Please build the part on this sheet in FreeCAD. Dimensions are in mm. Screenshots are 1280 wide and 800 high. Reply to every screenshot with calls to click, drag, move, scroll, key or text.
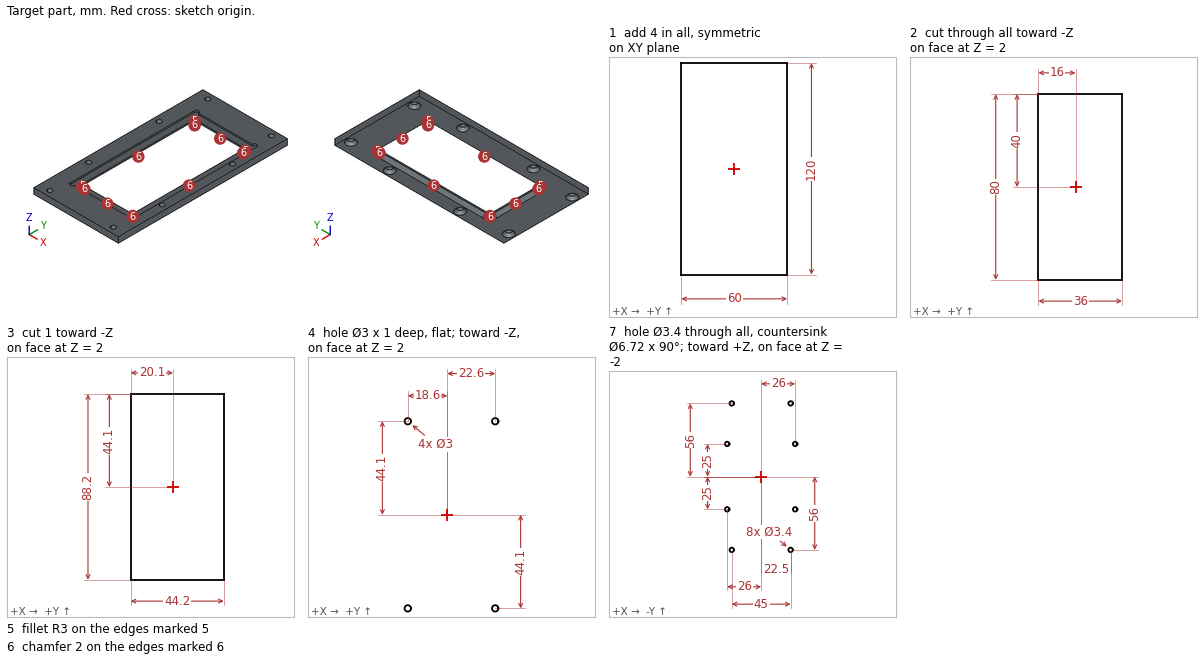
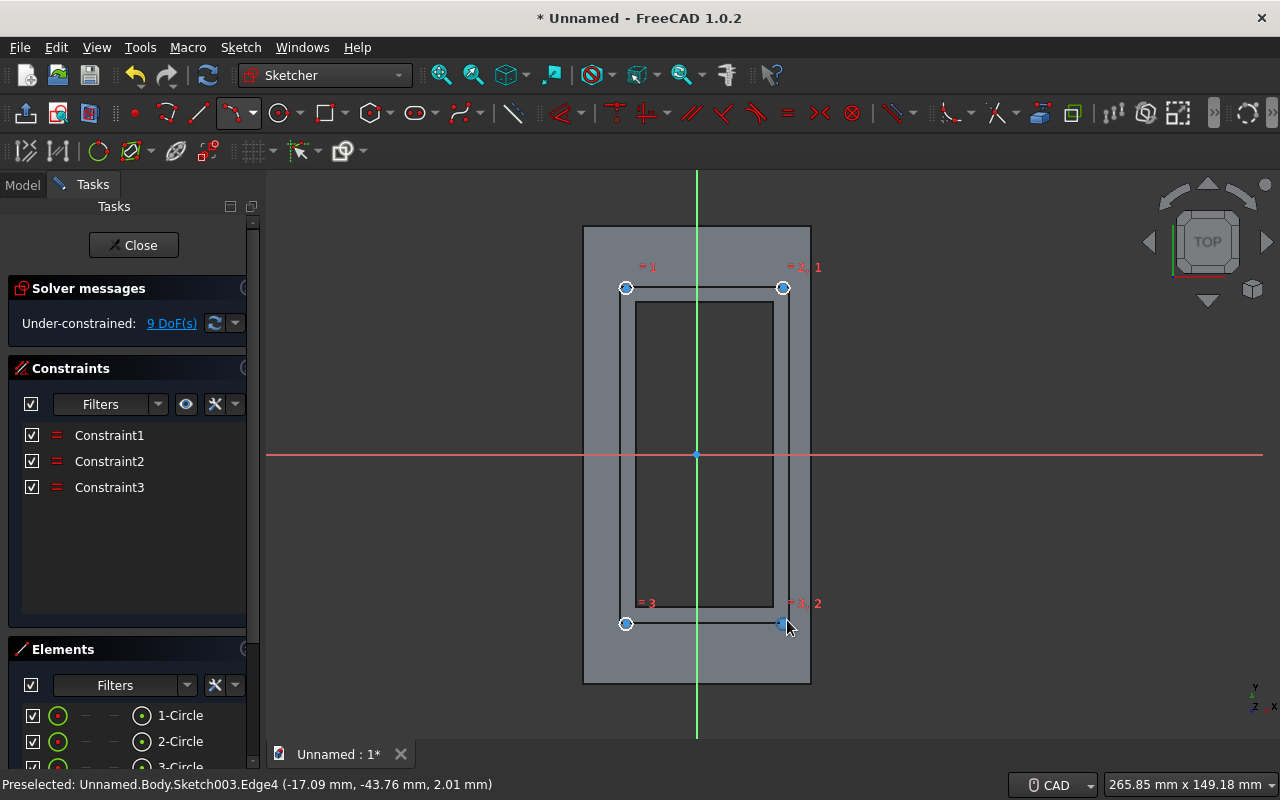
click(626, 288)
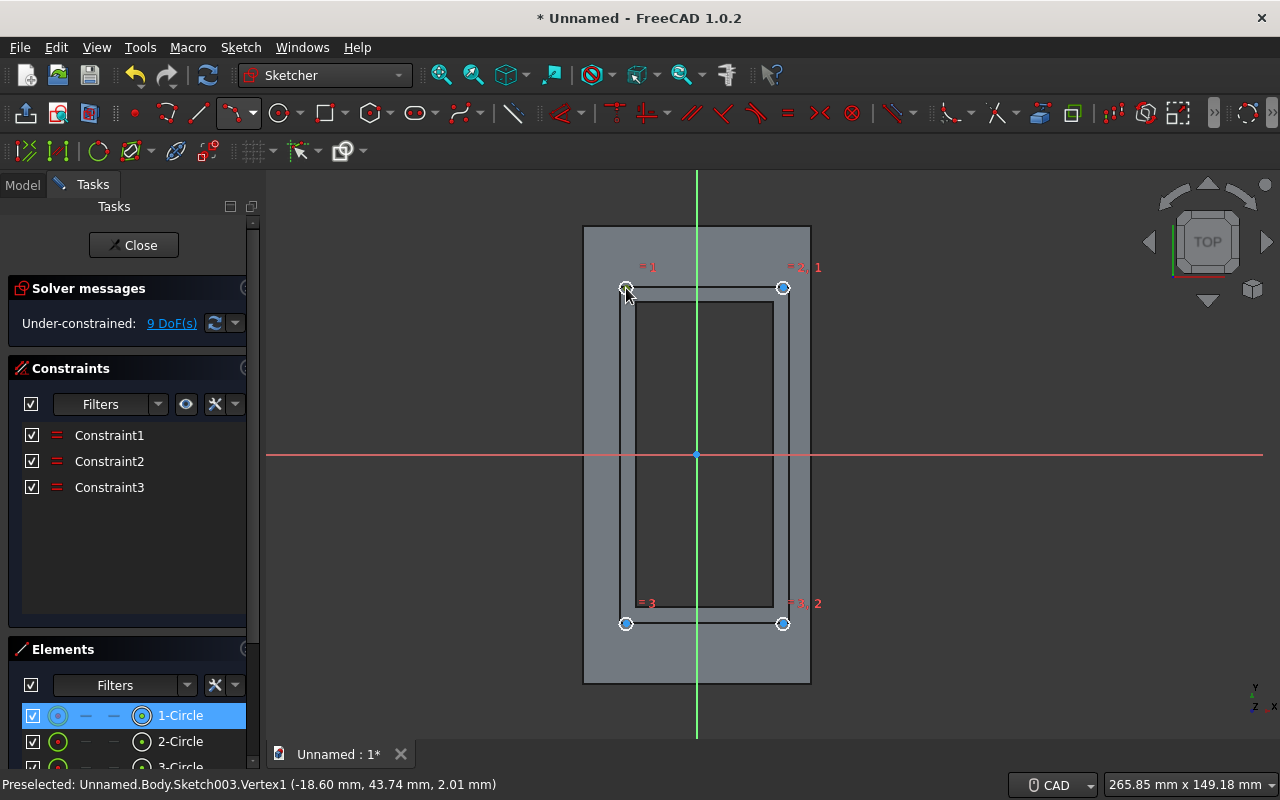
click(783, 288)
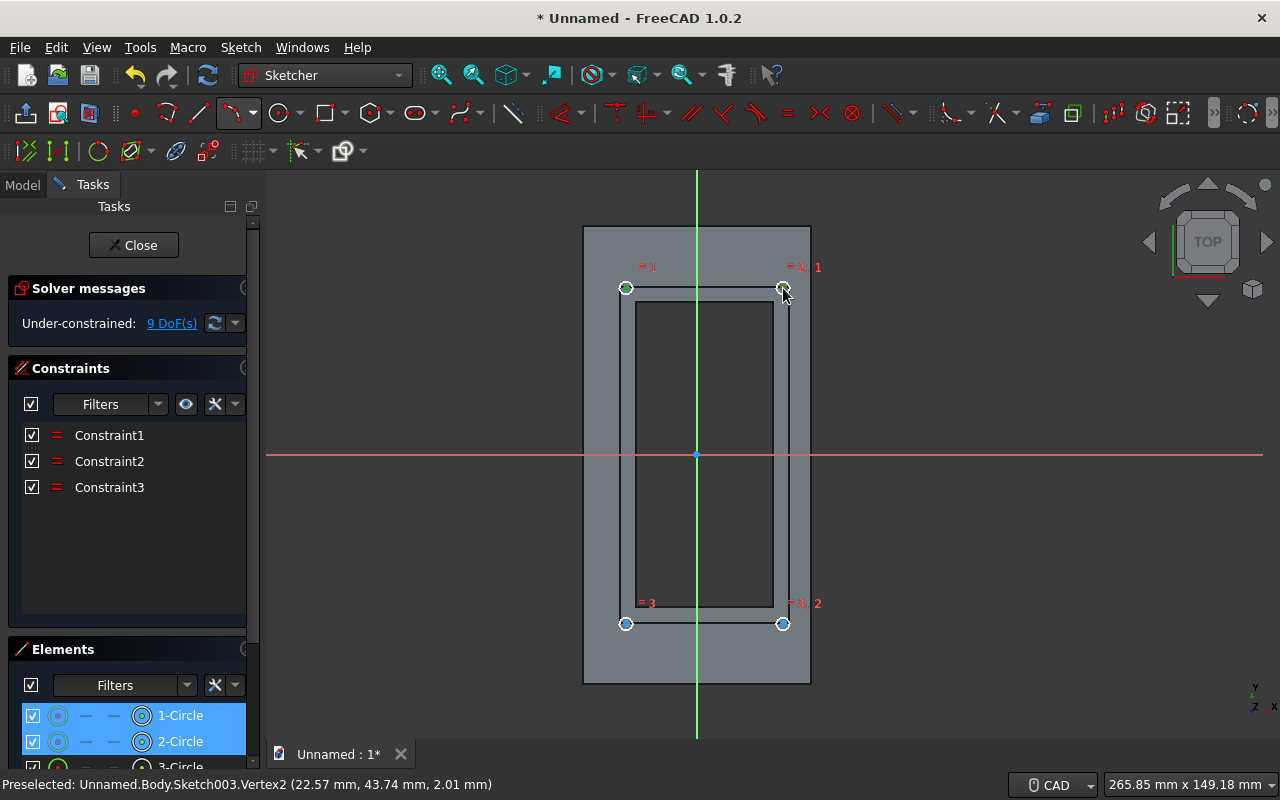
click(670, 114)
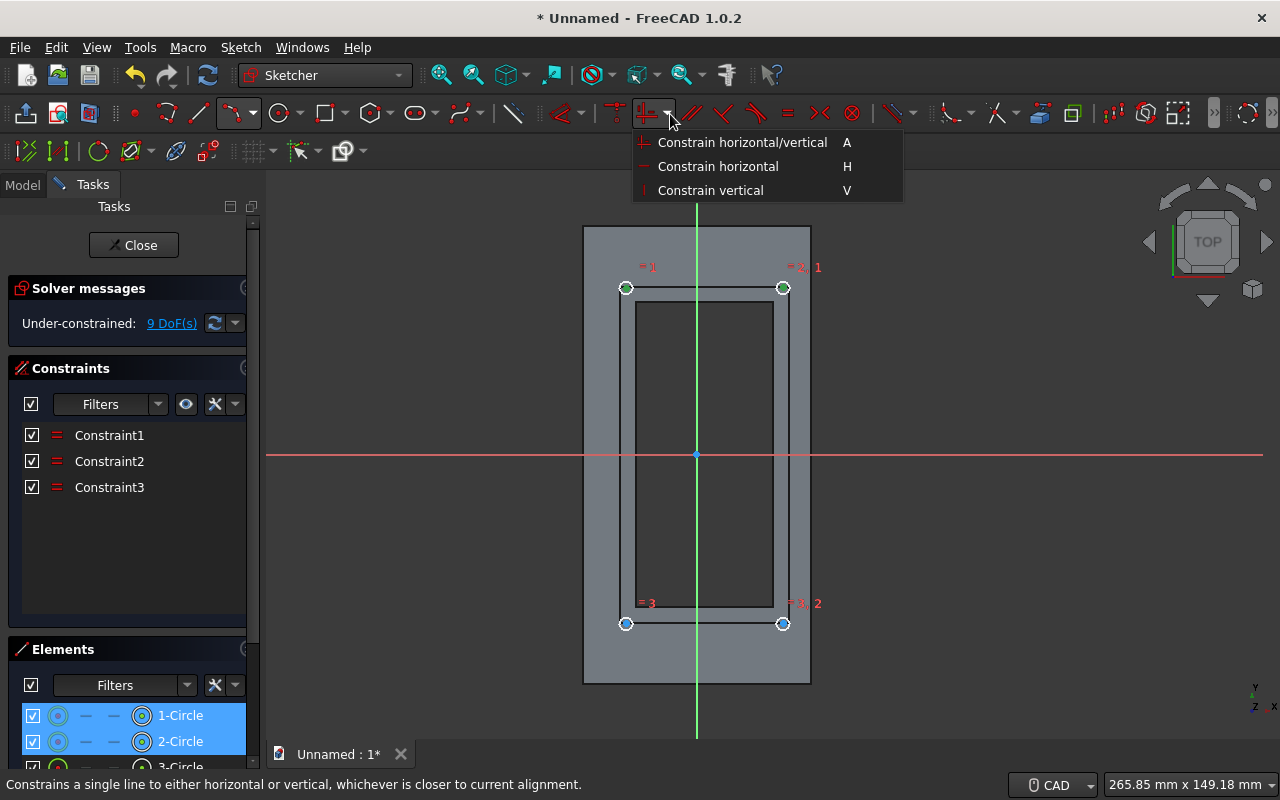
click(768, 166)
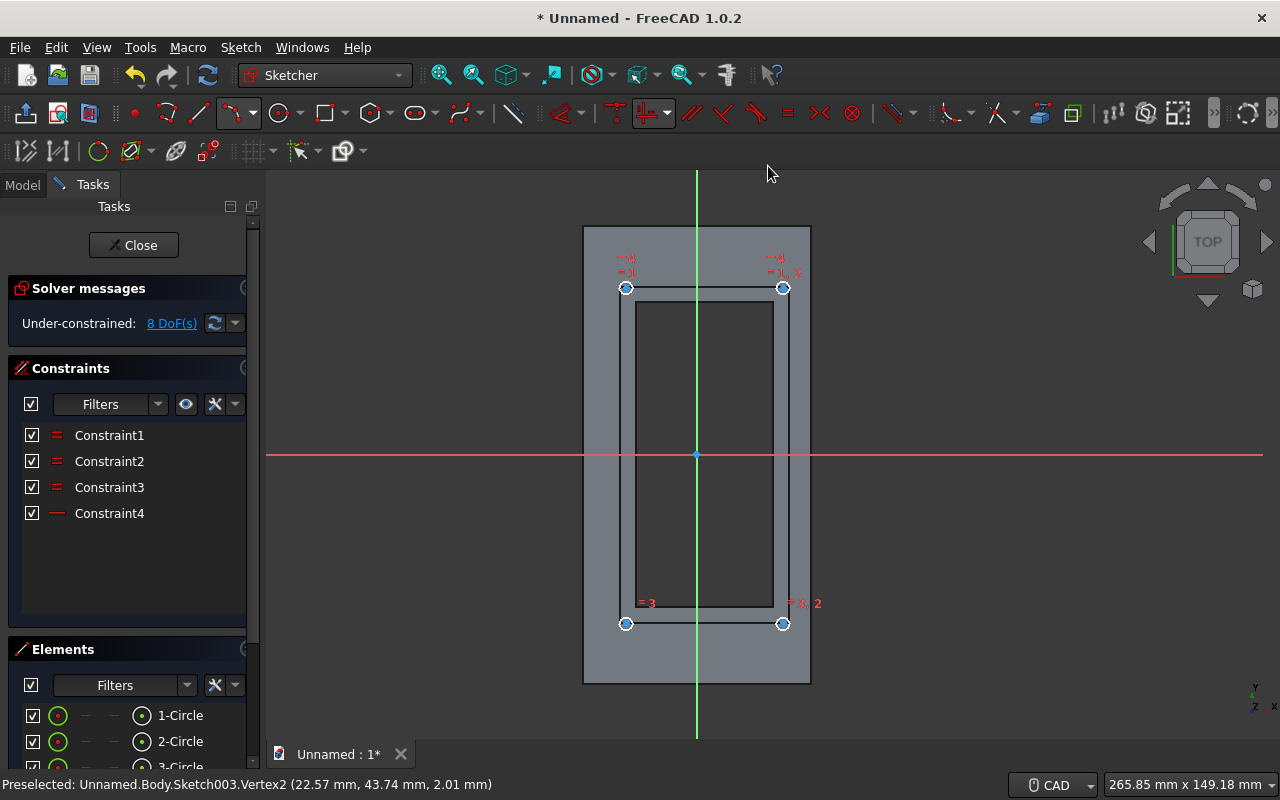
click(783, 288)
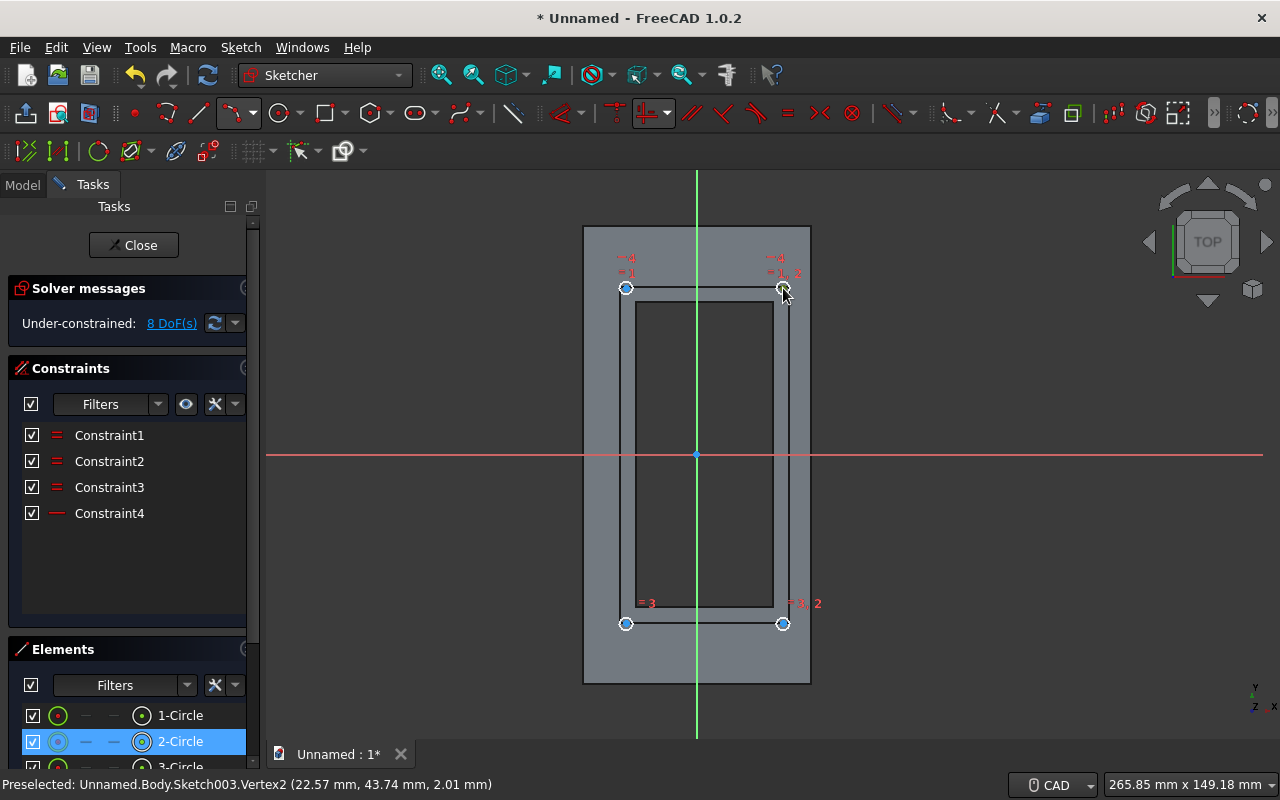
click(783, 624)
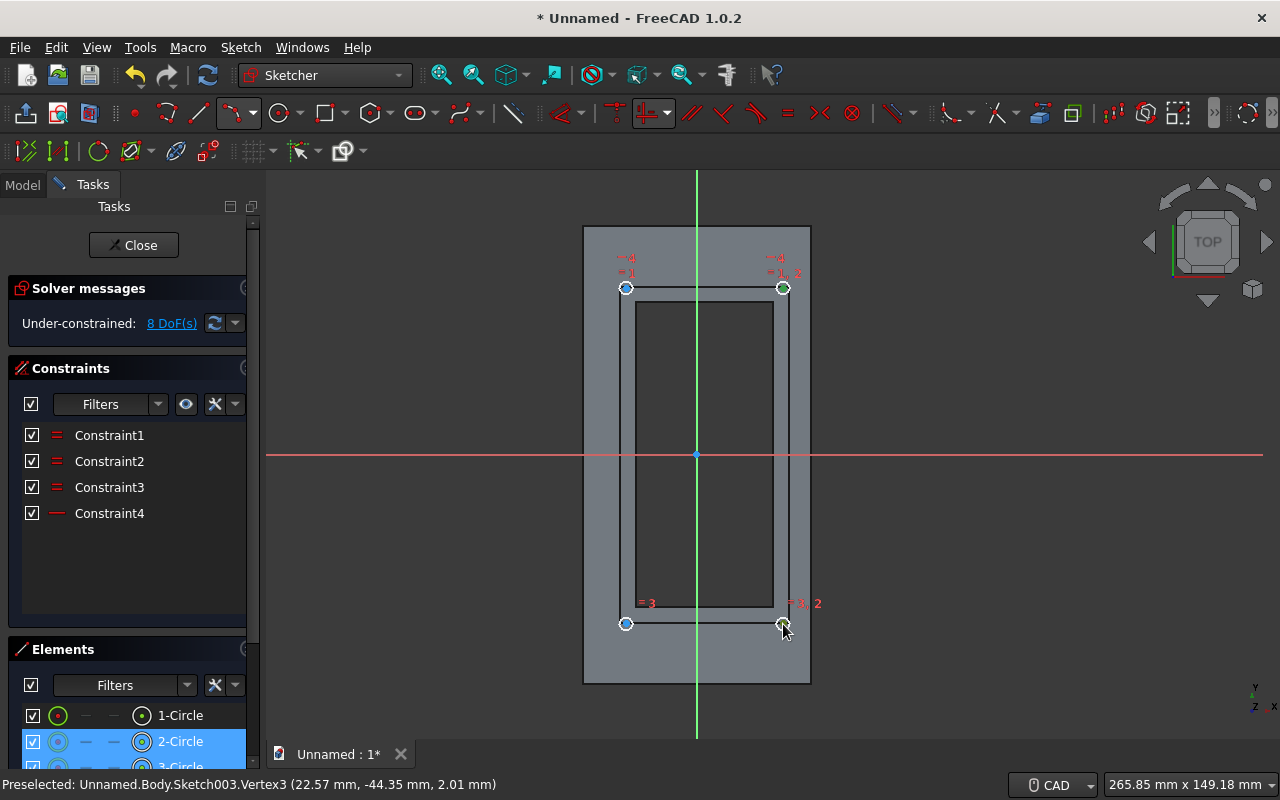
key(v)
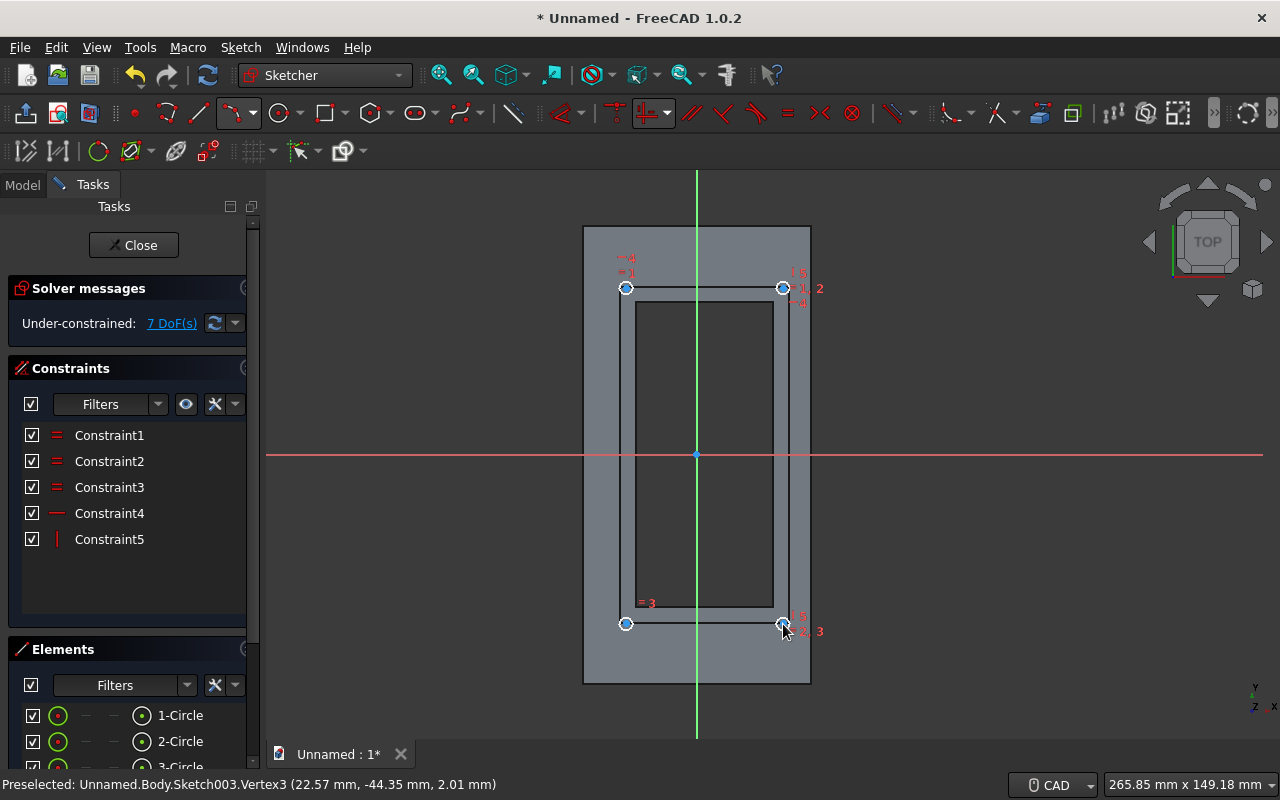
click(626, 288)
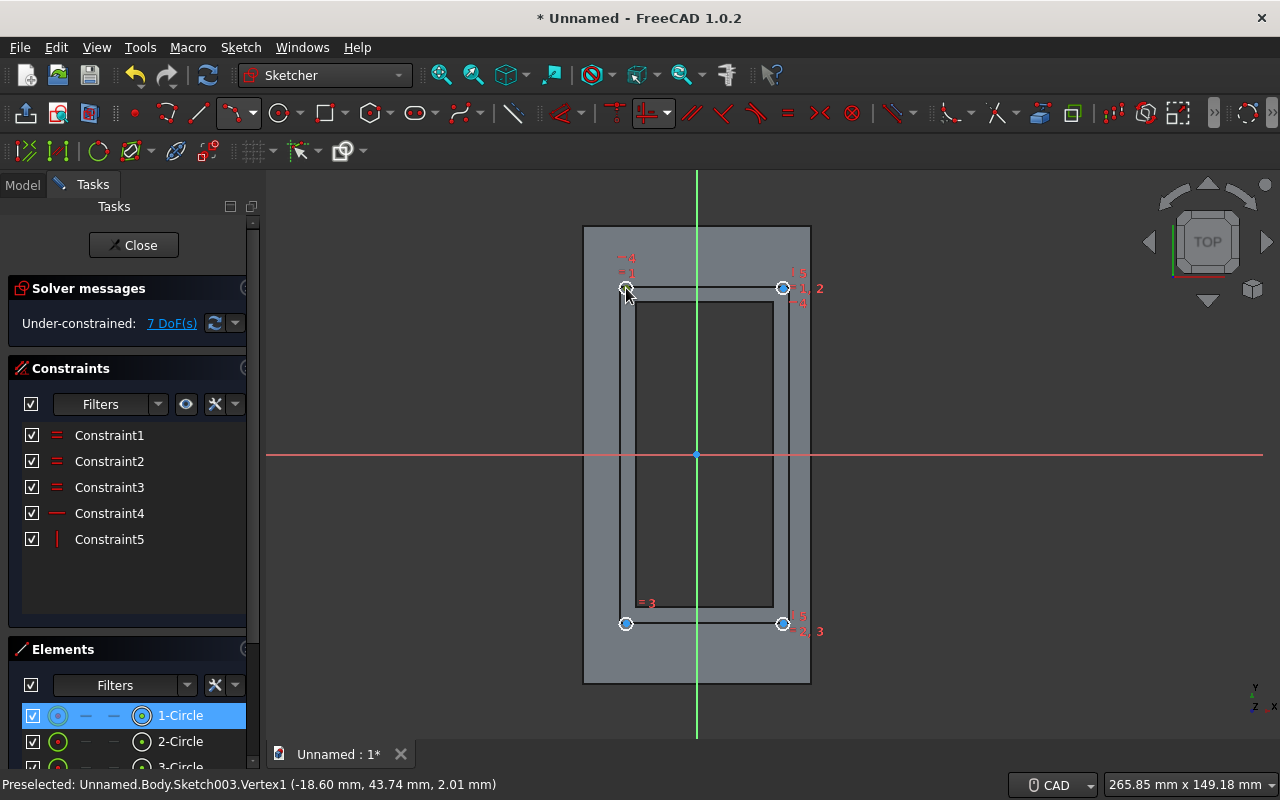
click(626, 624)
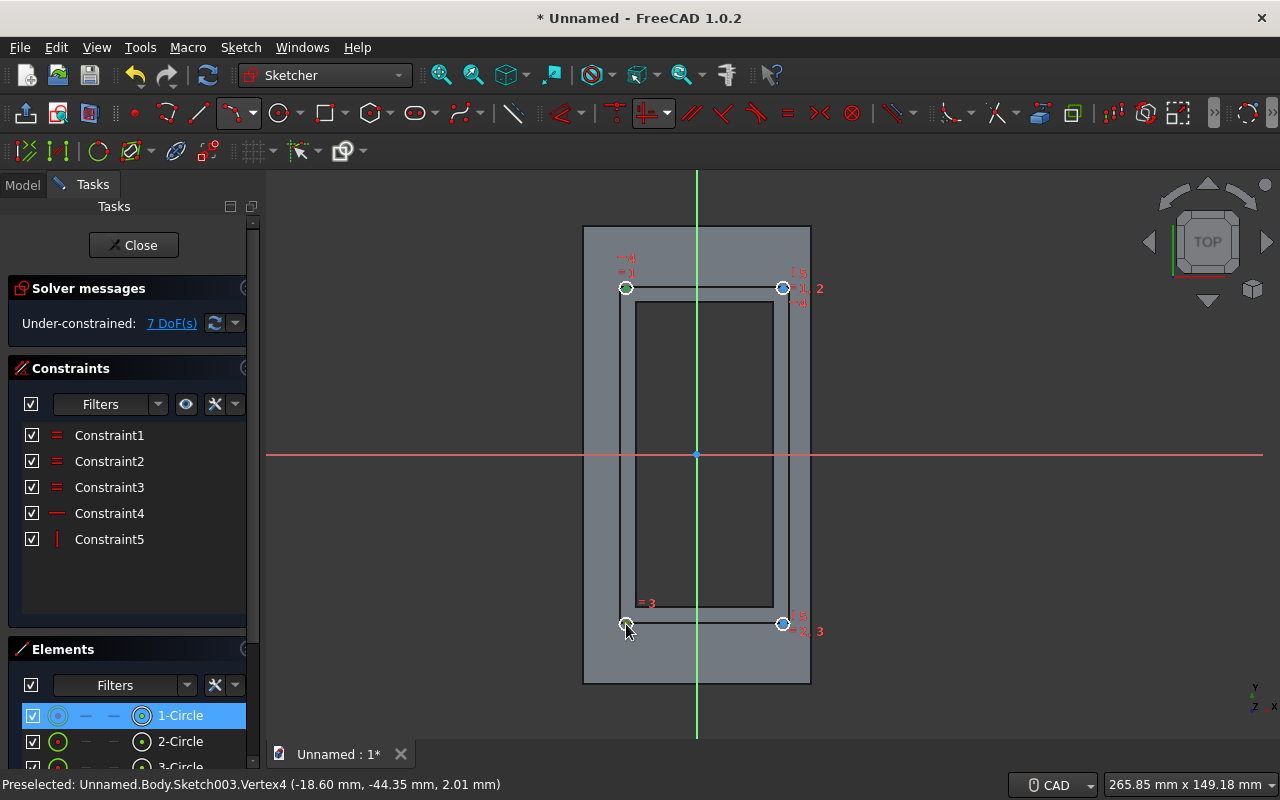
key(v)